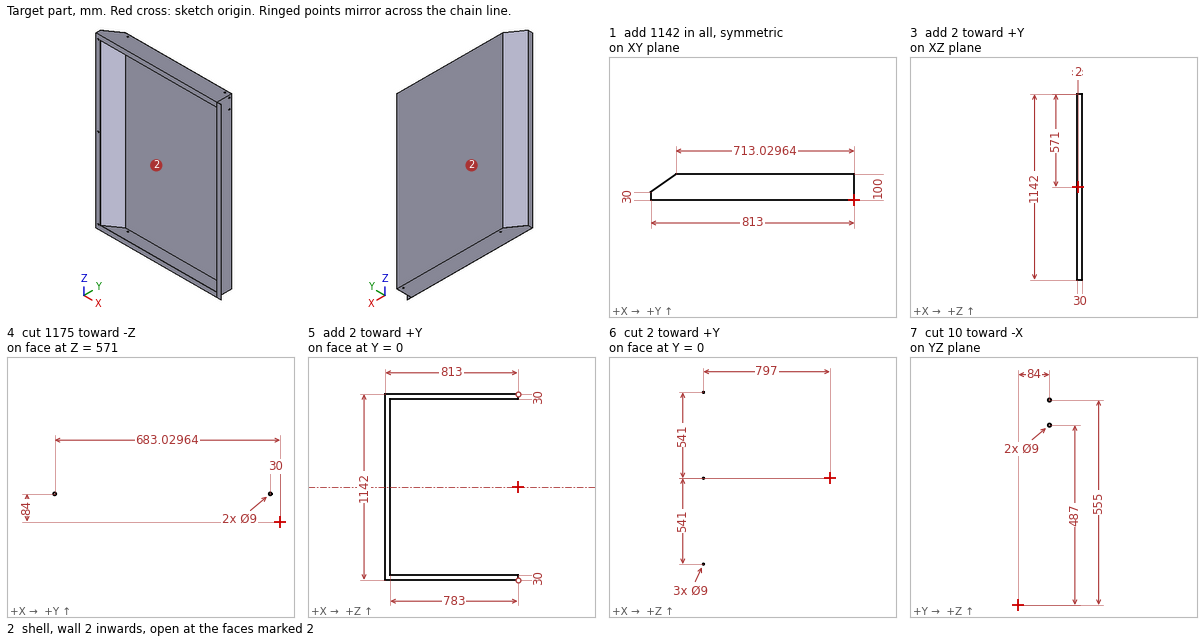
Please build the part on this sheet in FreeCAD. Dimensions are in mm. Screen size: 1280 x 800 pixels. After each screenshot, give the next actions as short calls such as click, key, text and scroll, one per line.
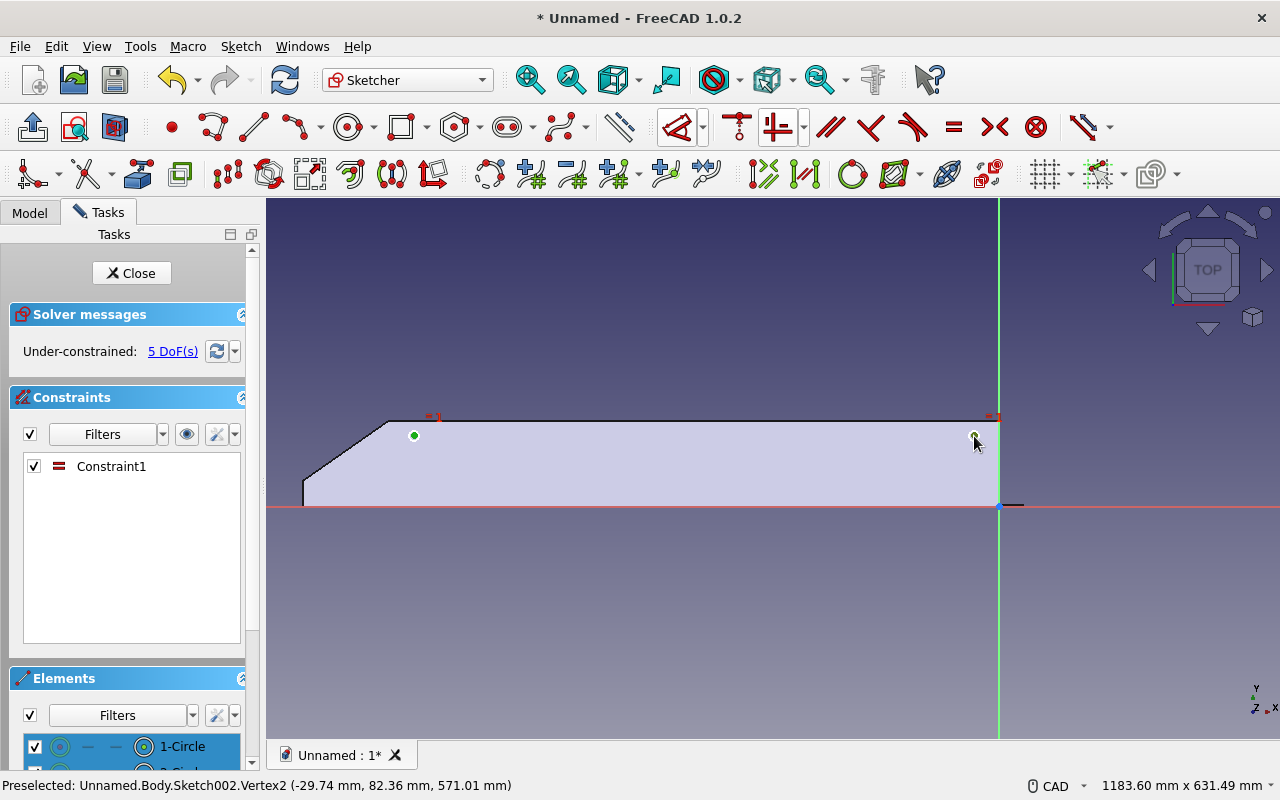
click(804, 128)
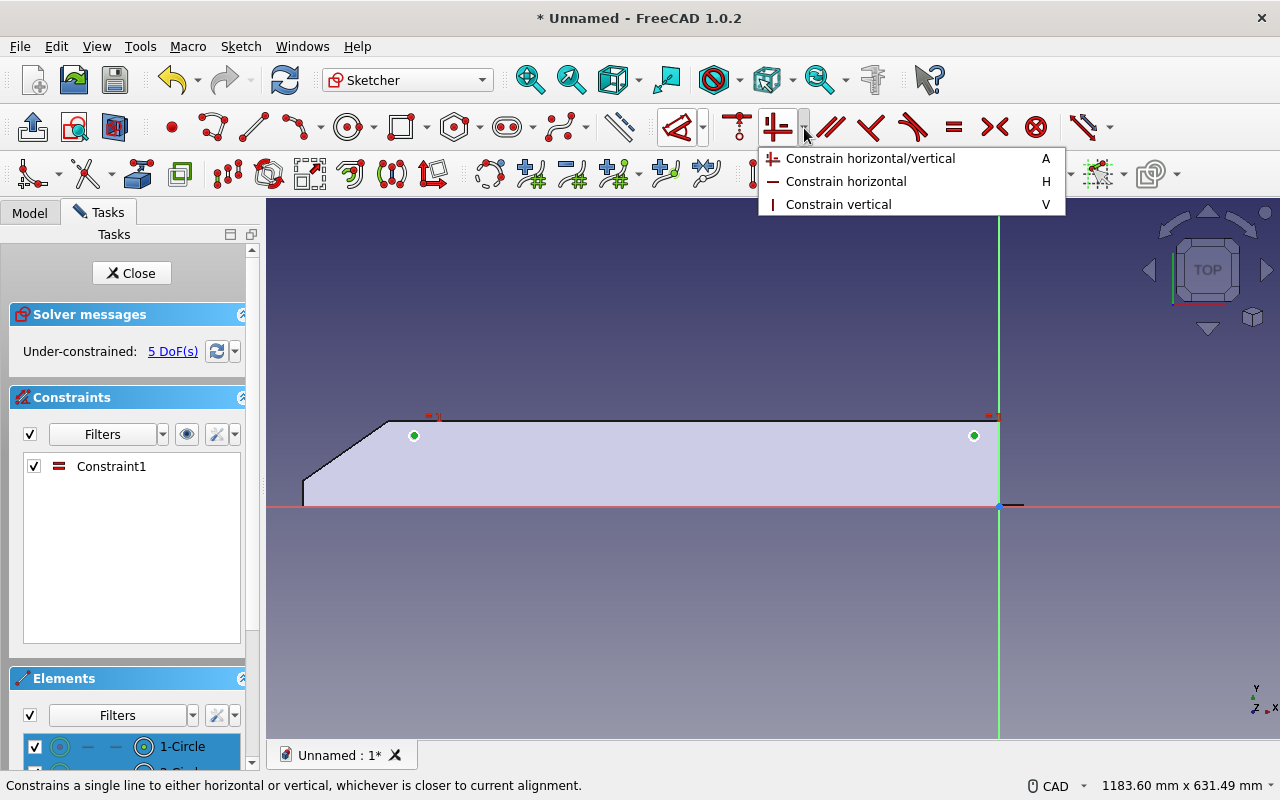
click(912, 182)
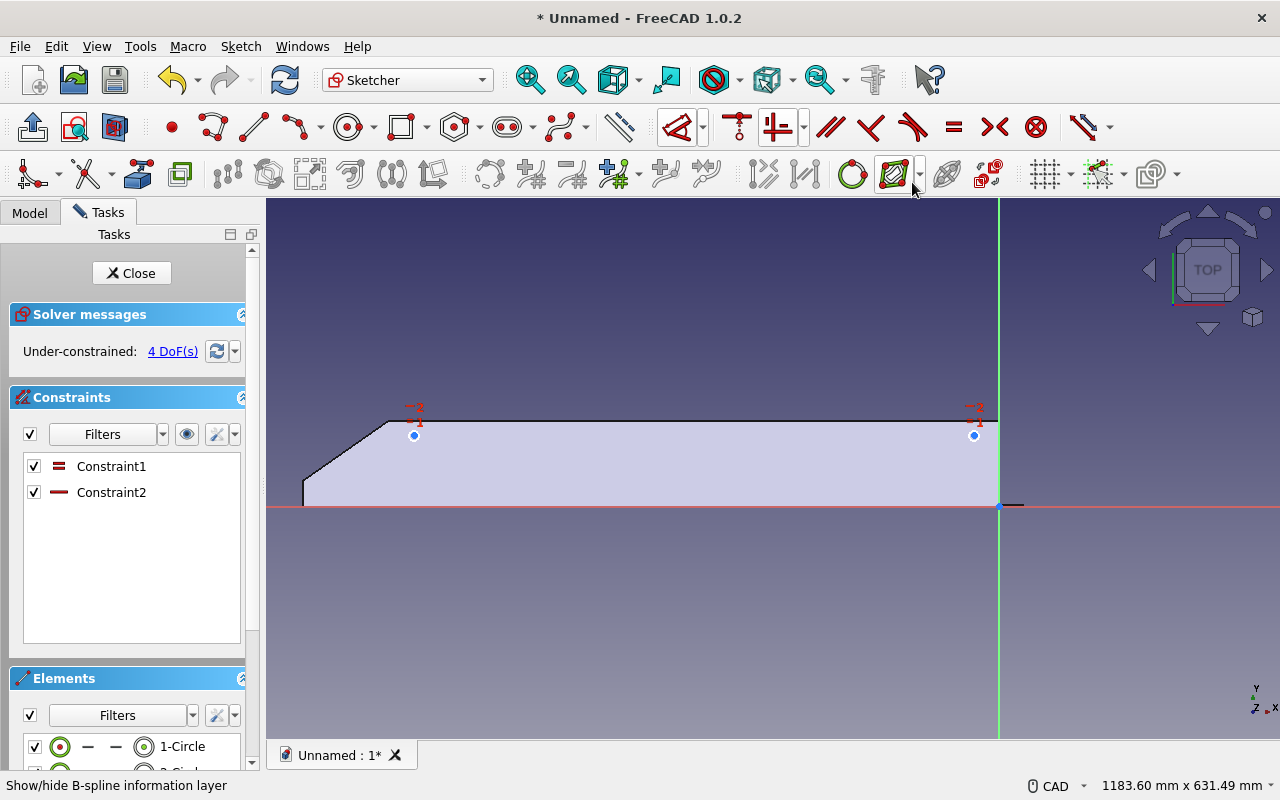
scroll(417, 432, up, 9)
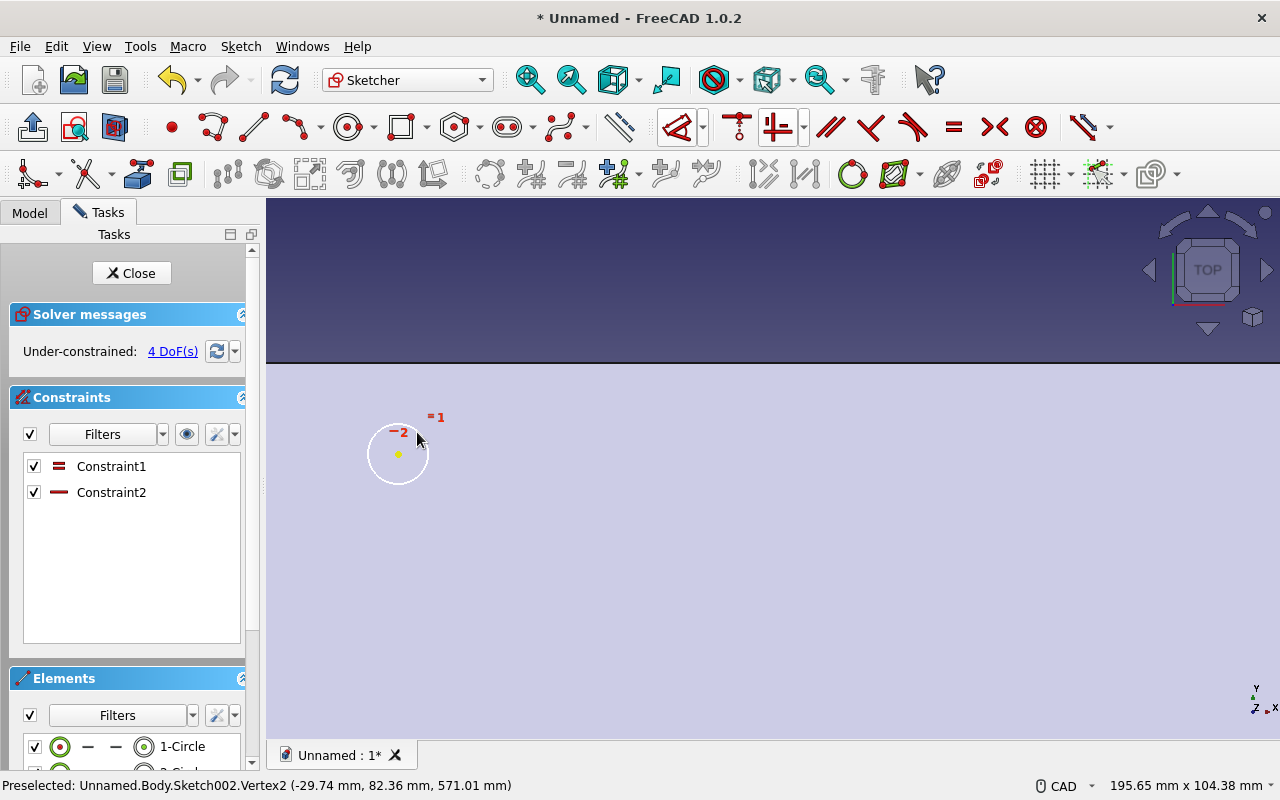
click(419, 433)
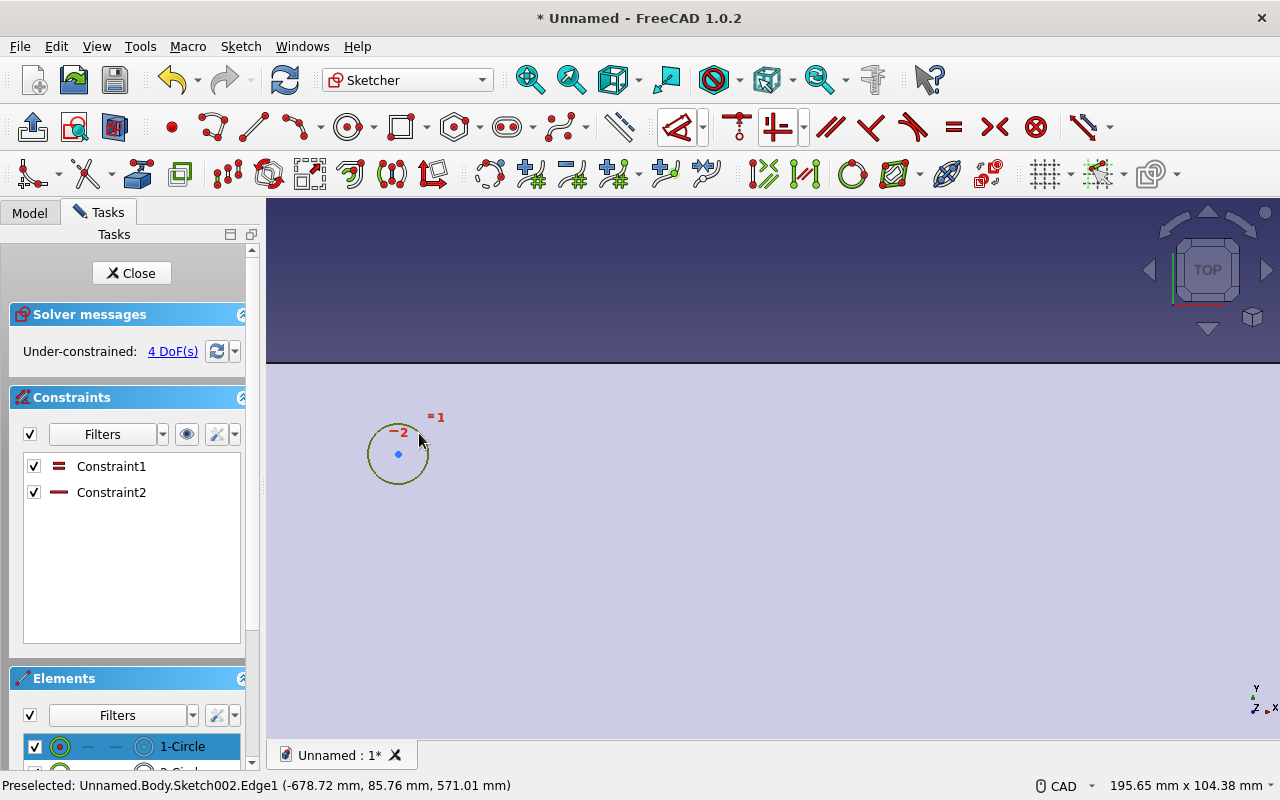
click(702, 128)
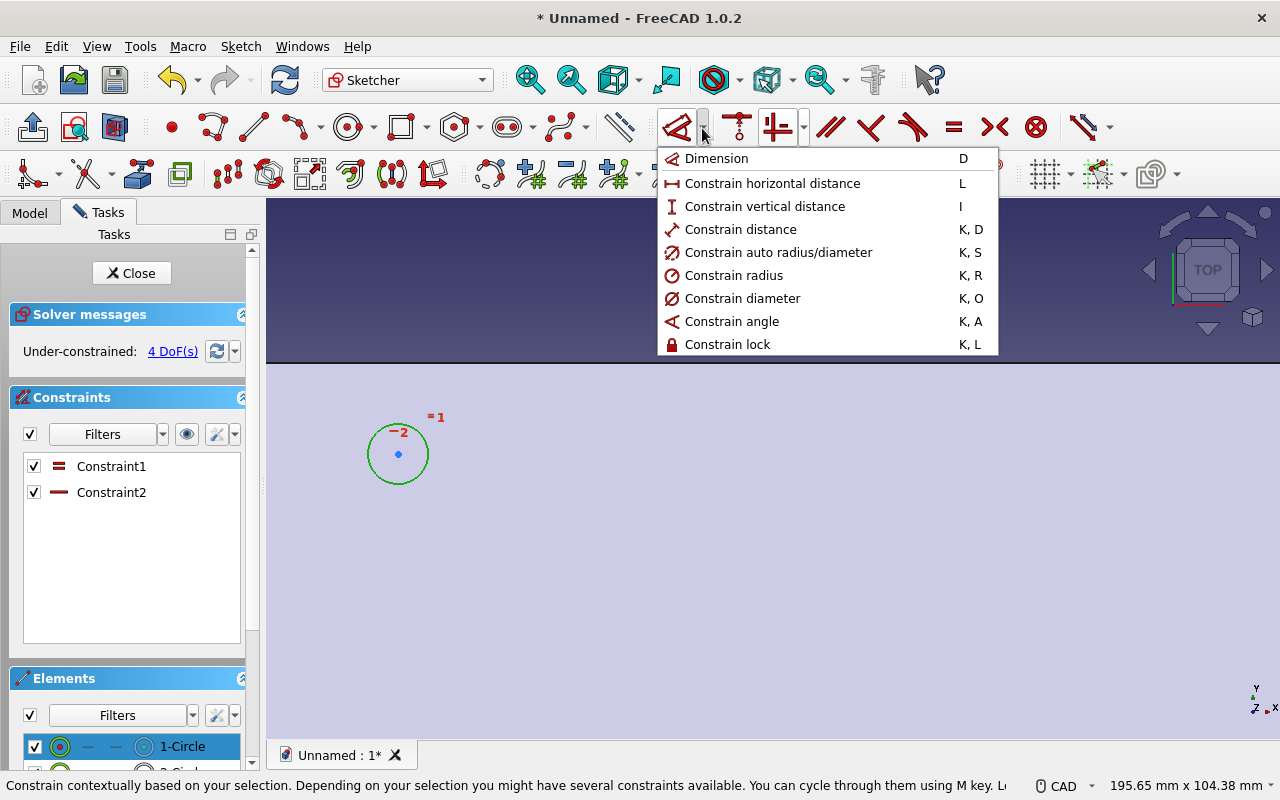
click(828, 298)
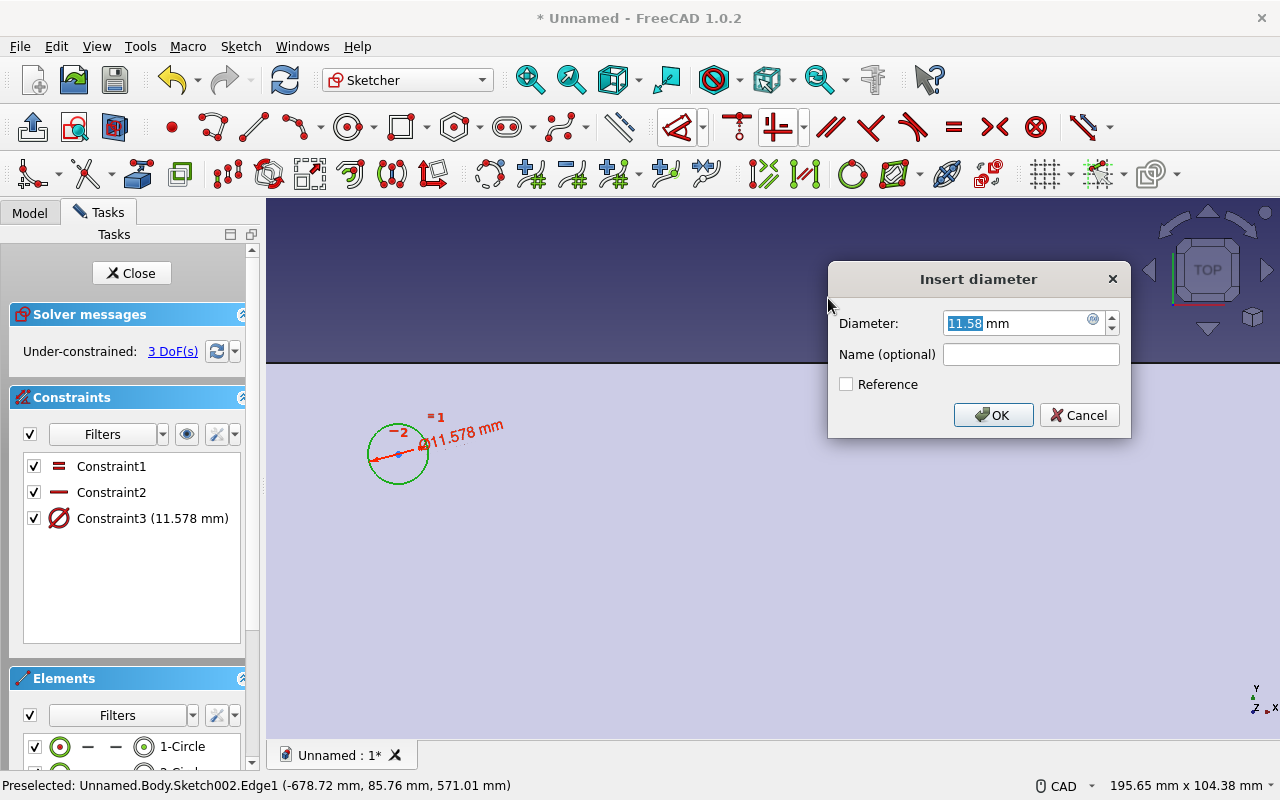
text(9)
key(Return)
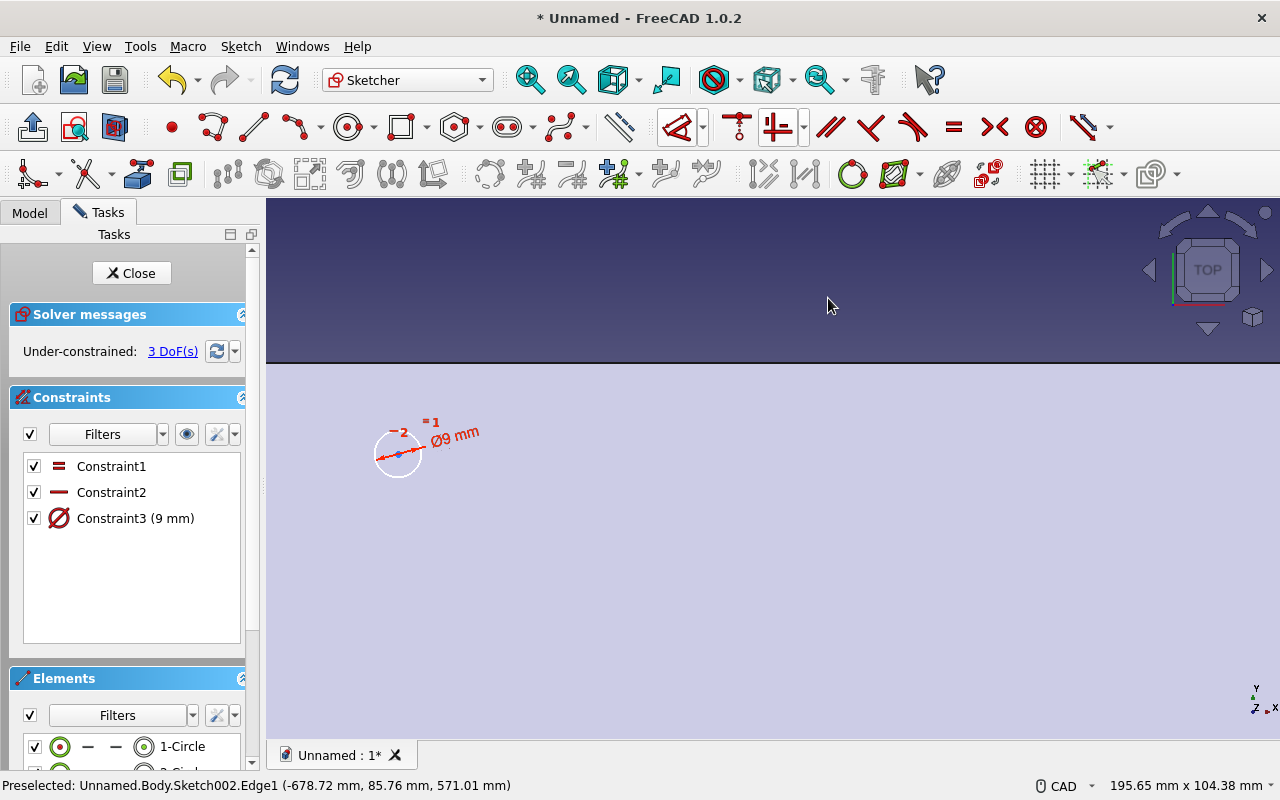
scroll(417, 432, down, 9)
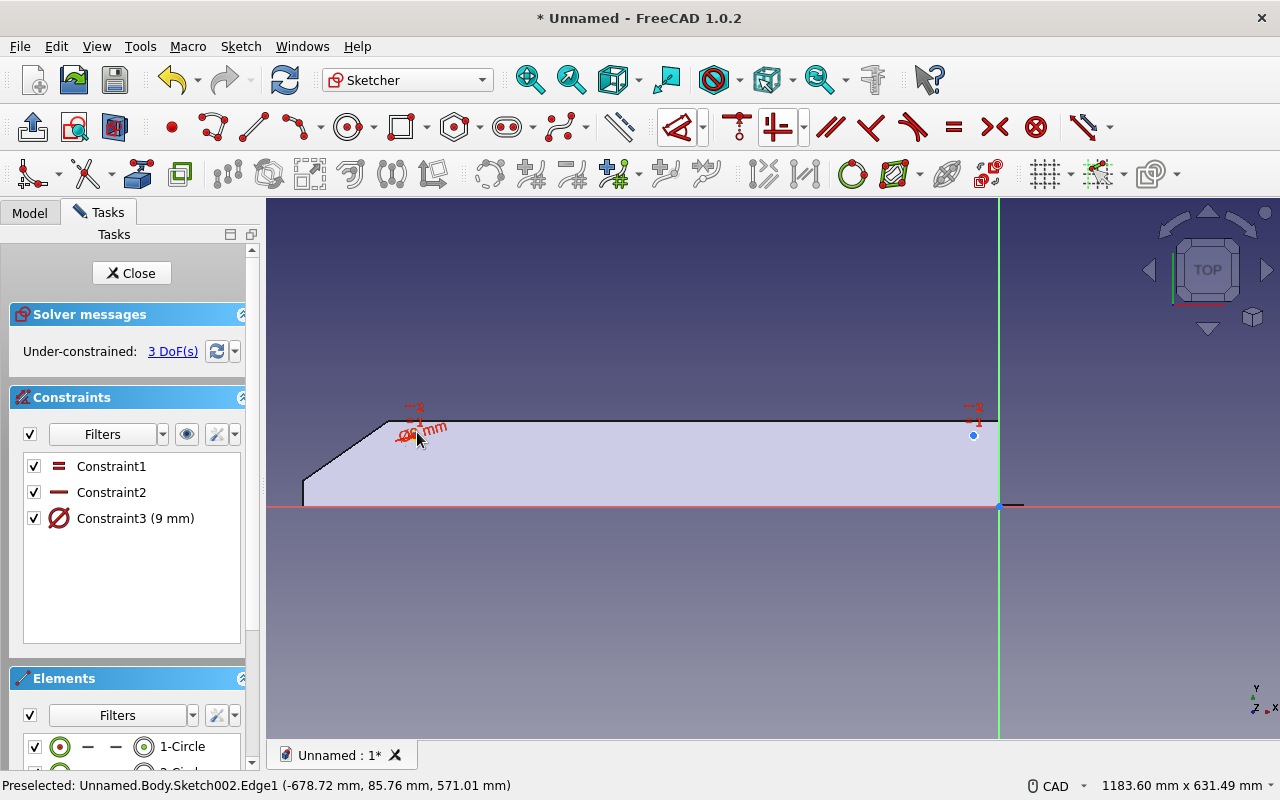
click(414, 436)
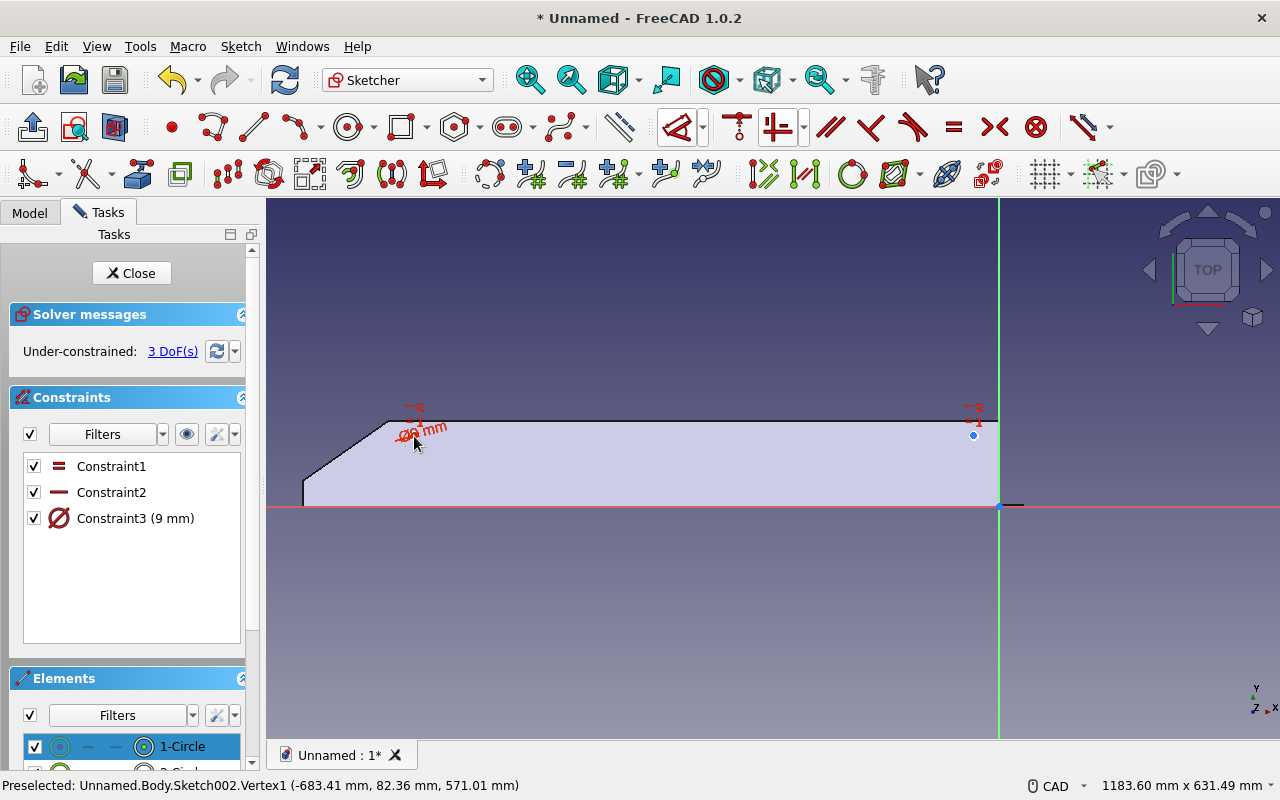
click(702, 128)